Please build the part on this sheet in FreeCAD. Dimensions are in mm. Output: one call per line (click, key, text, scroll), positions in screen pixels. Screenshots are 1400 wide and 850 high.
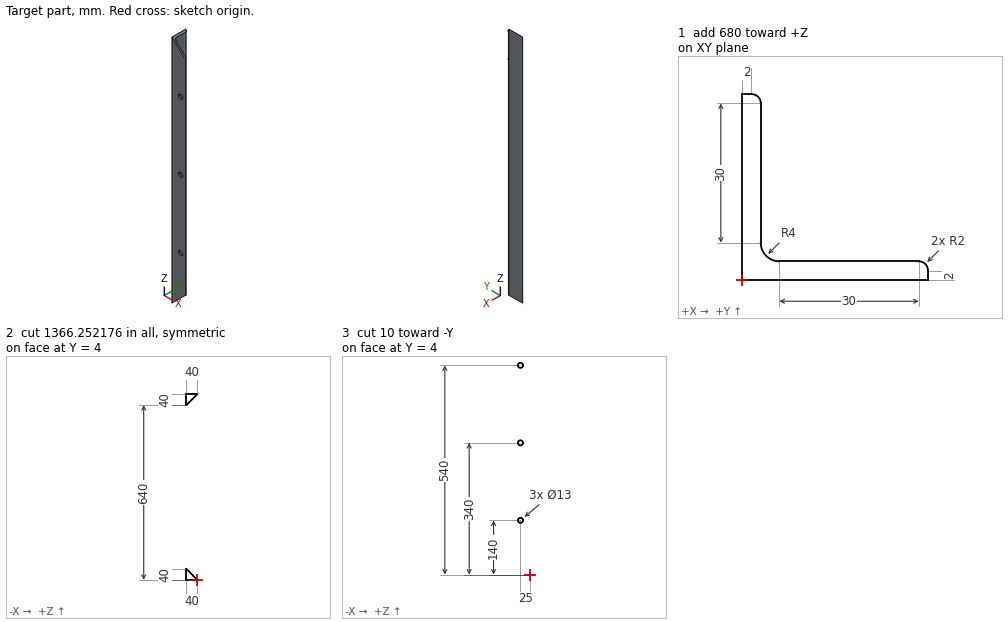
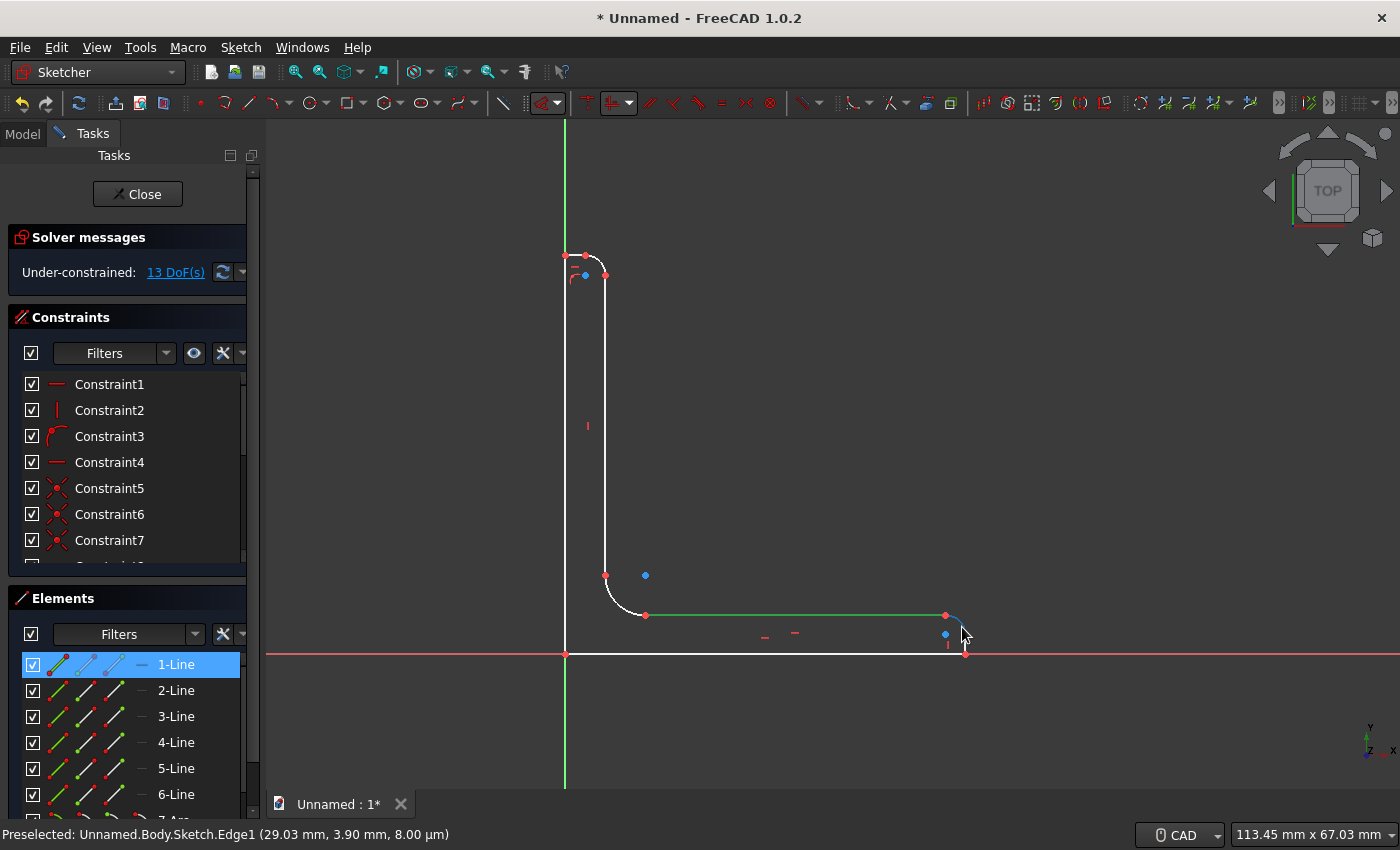
click(610, 593)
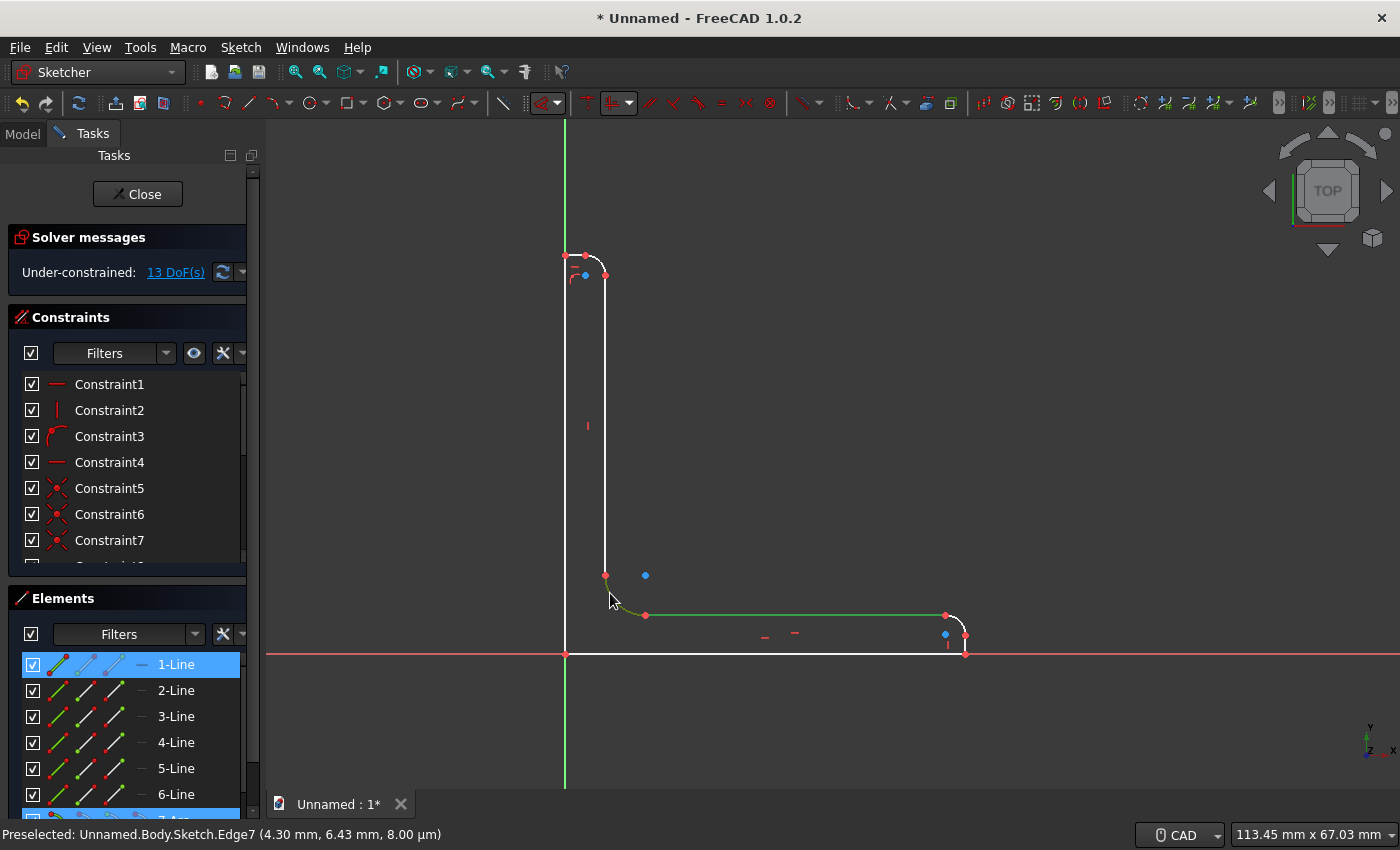
click(698, 104)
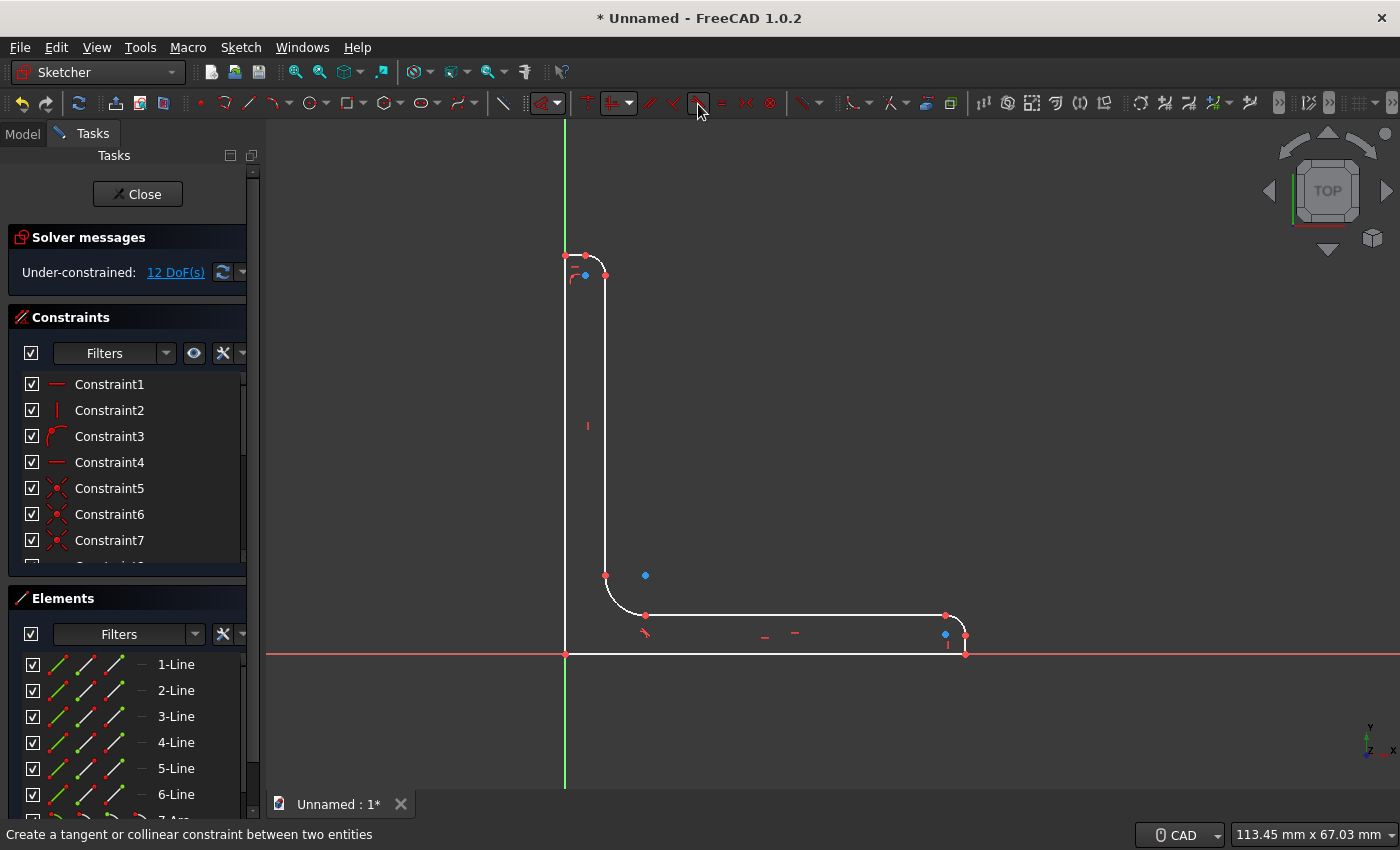
click(855, 615)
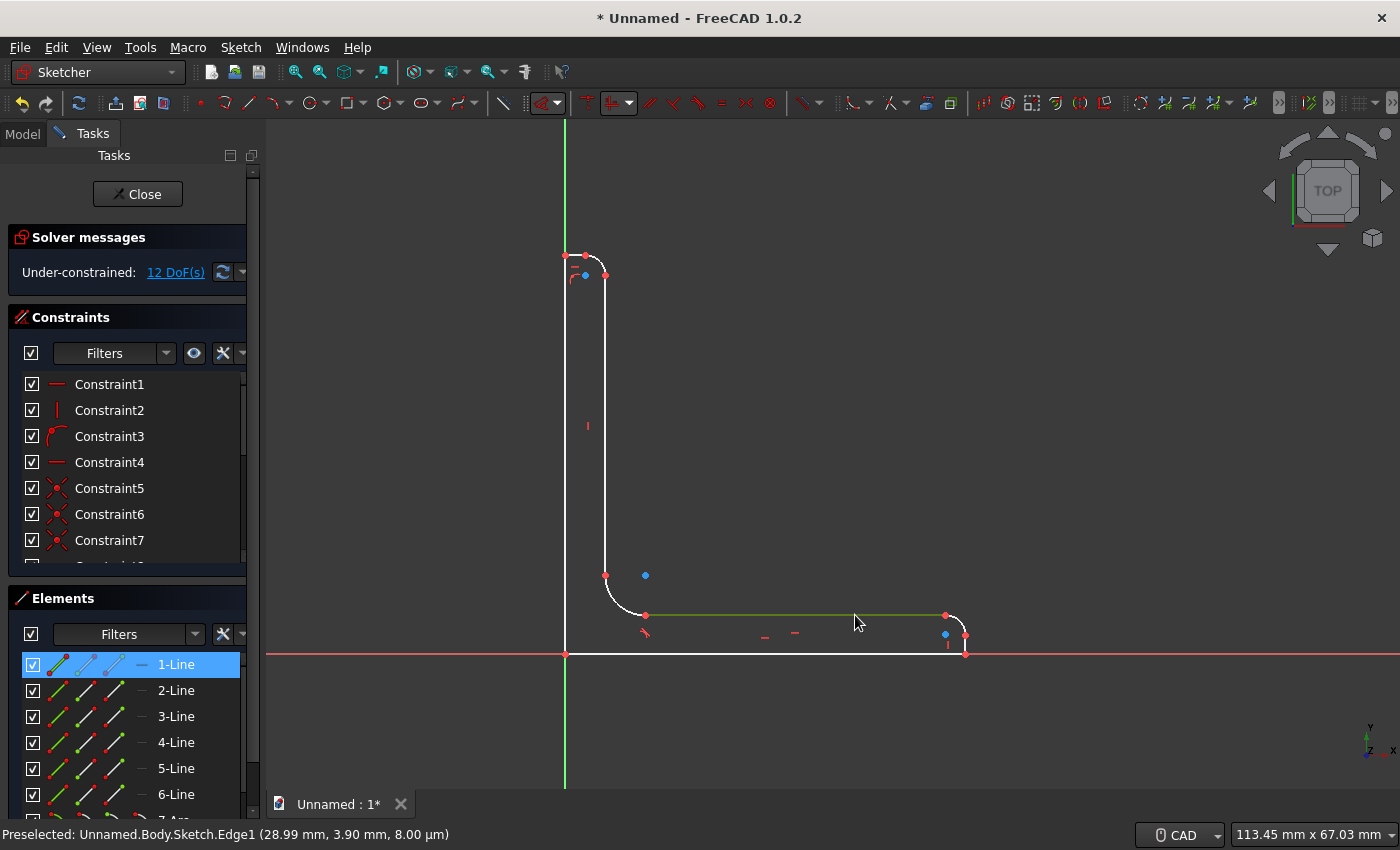
scroll(963, 626, up, 2)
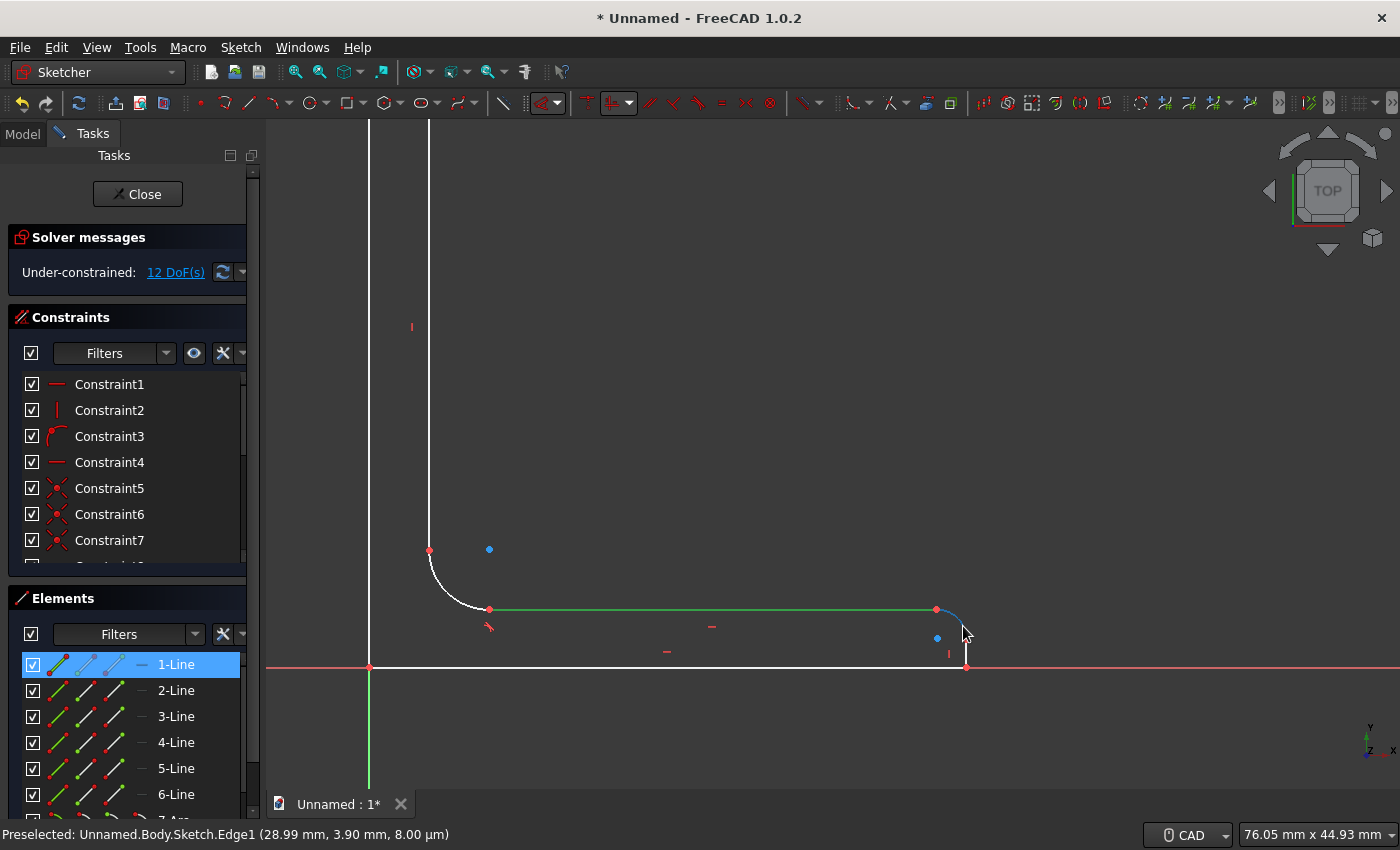
click(963, 626)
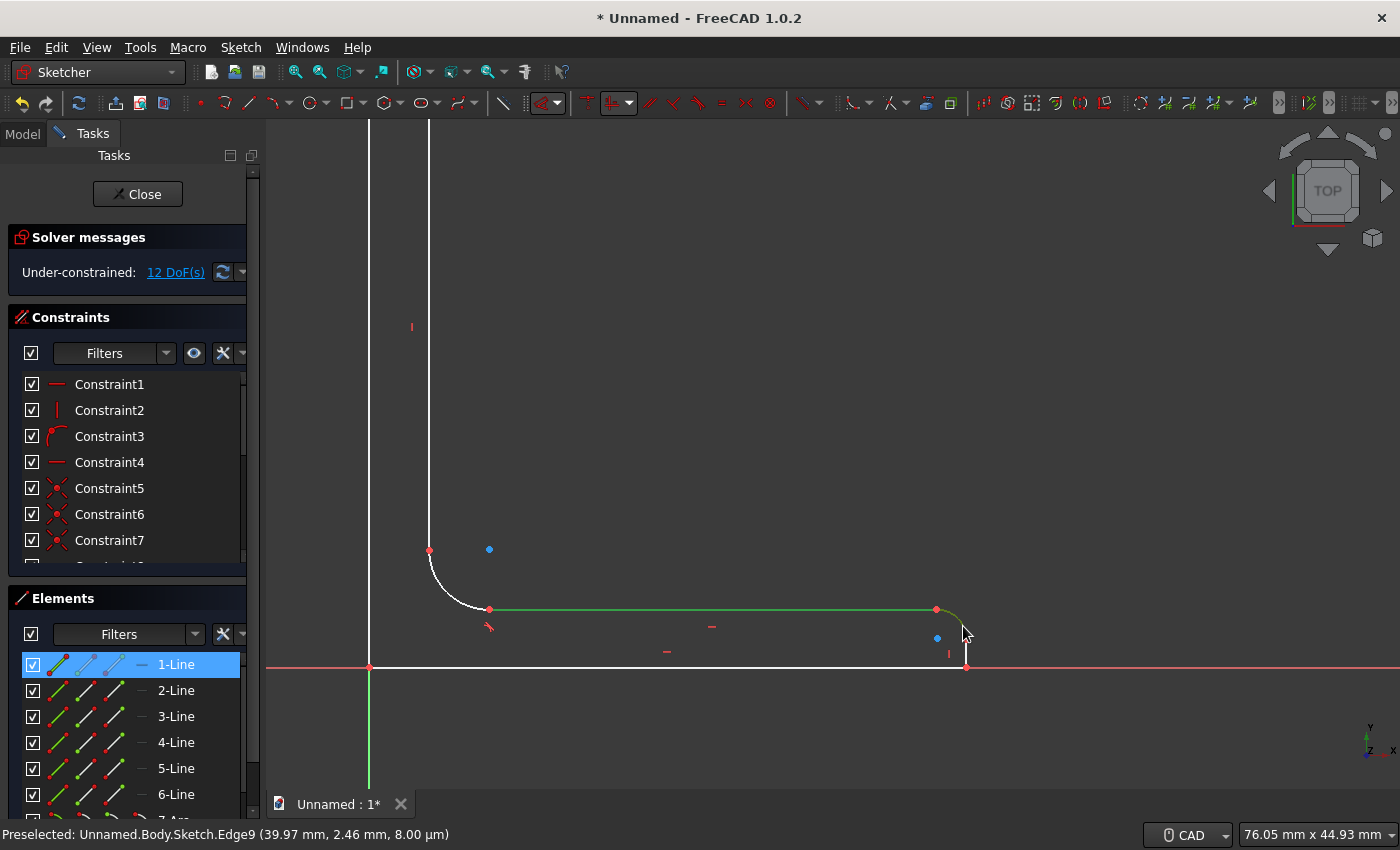
click(698, 104)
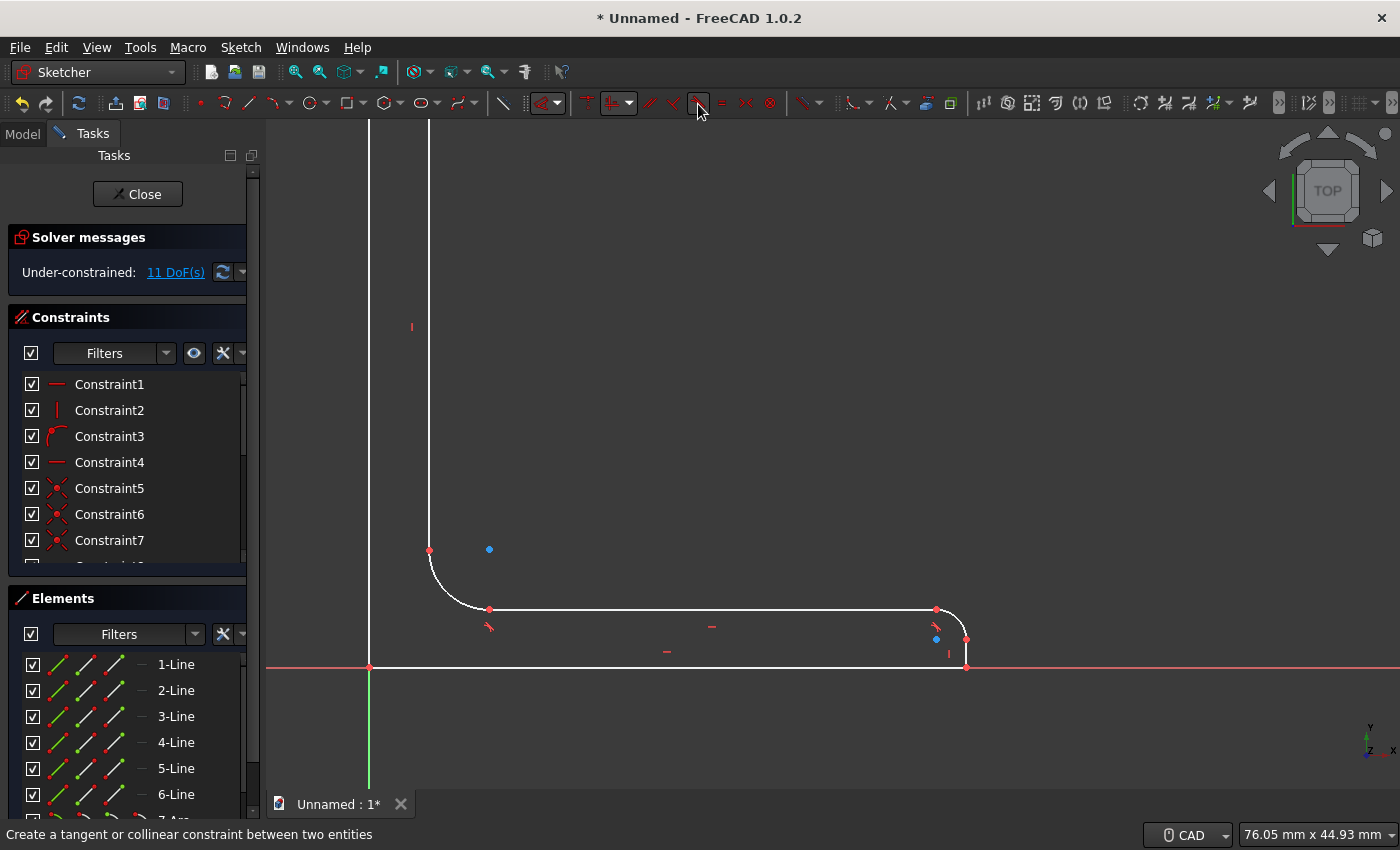
click(429, 416)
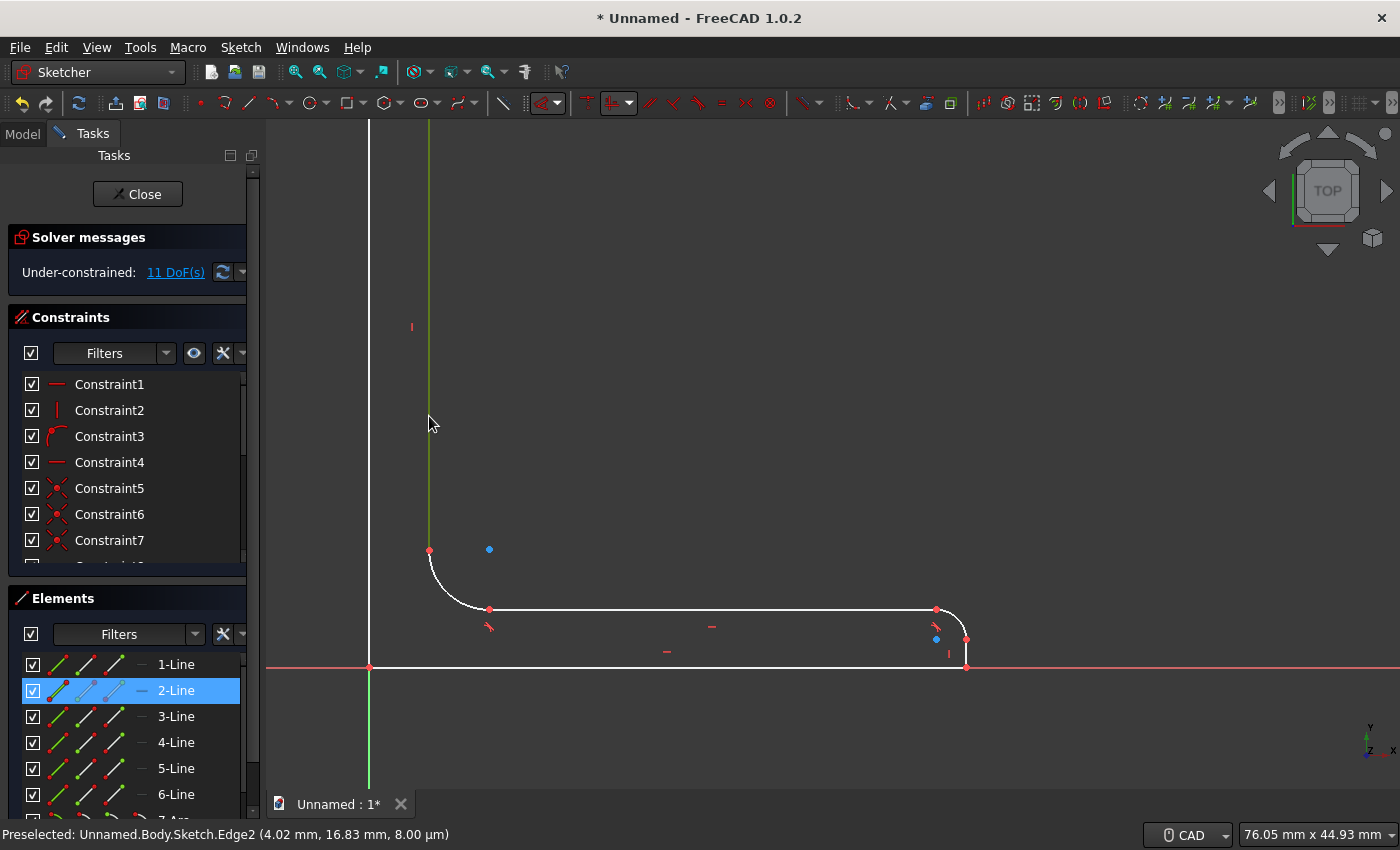
click(436, 577)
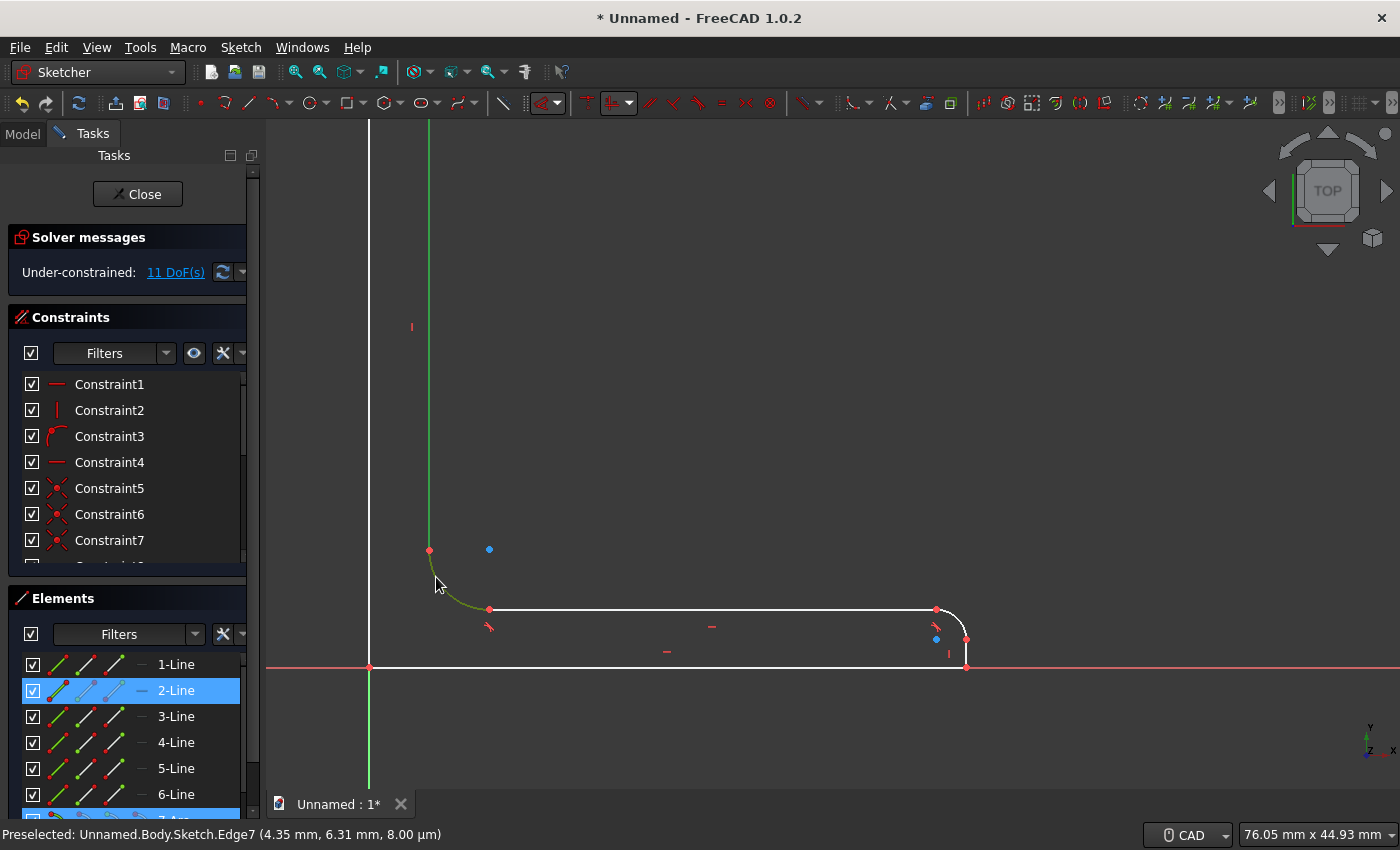
click(698, 104)